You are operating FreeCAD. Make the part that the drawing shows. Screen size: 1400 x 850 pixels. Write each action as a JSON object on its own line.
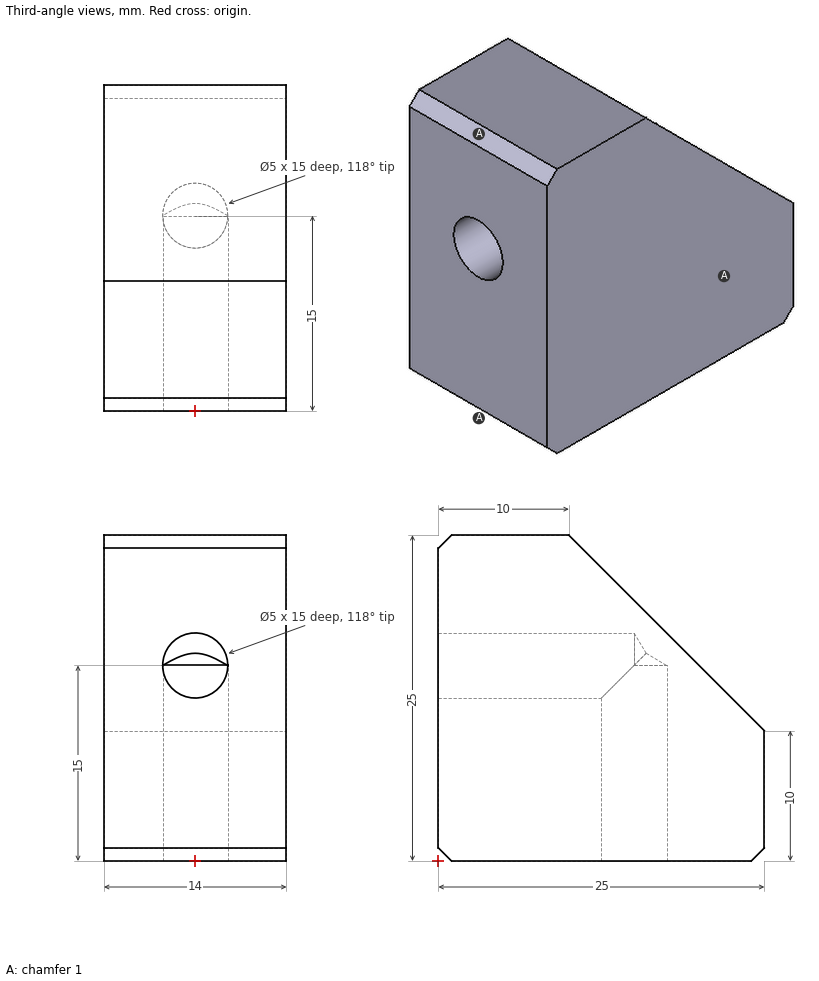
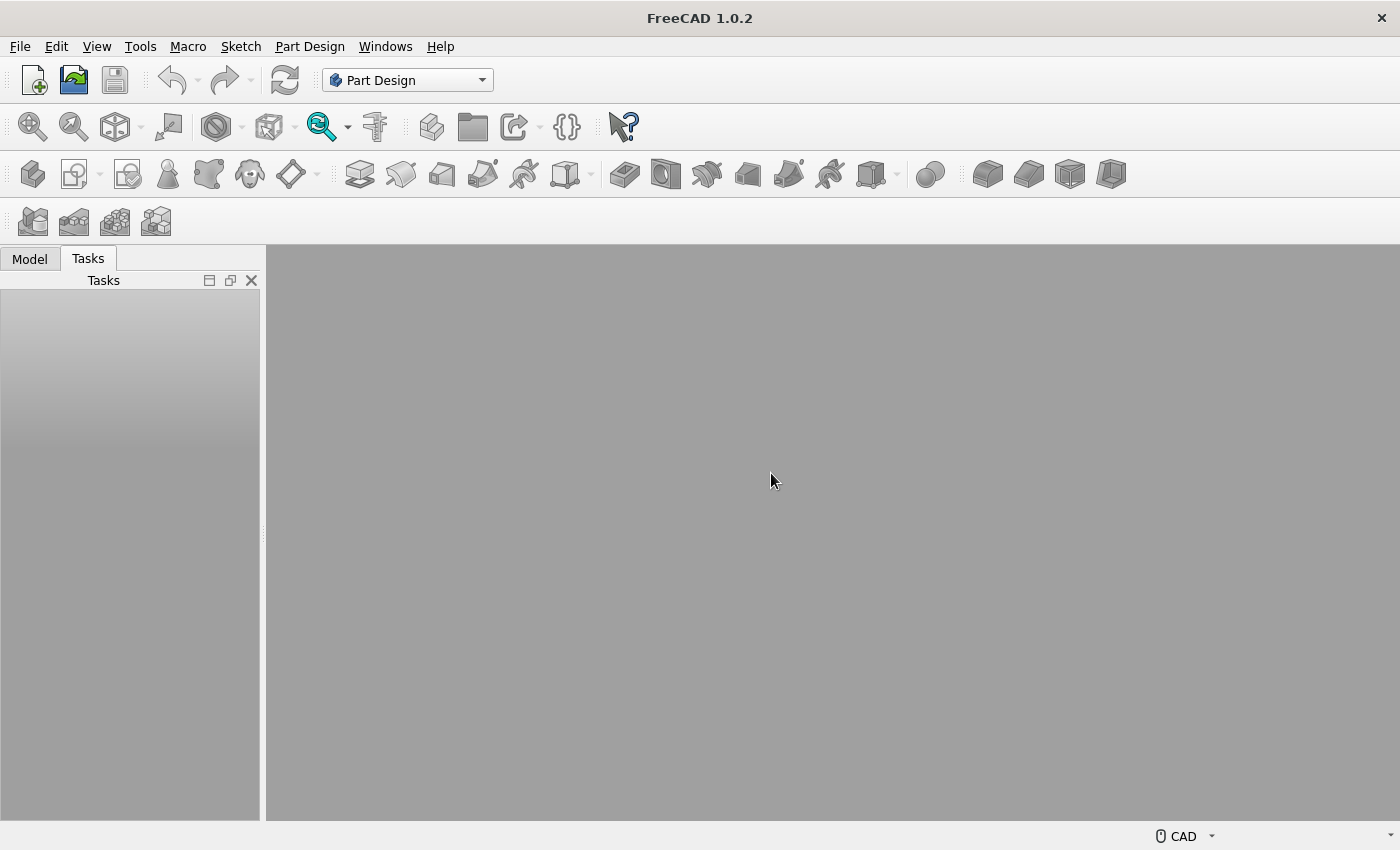
{"action": "left_click", "coordinate": [33, 80]}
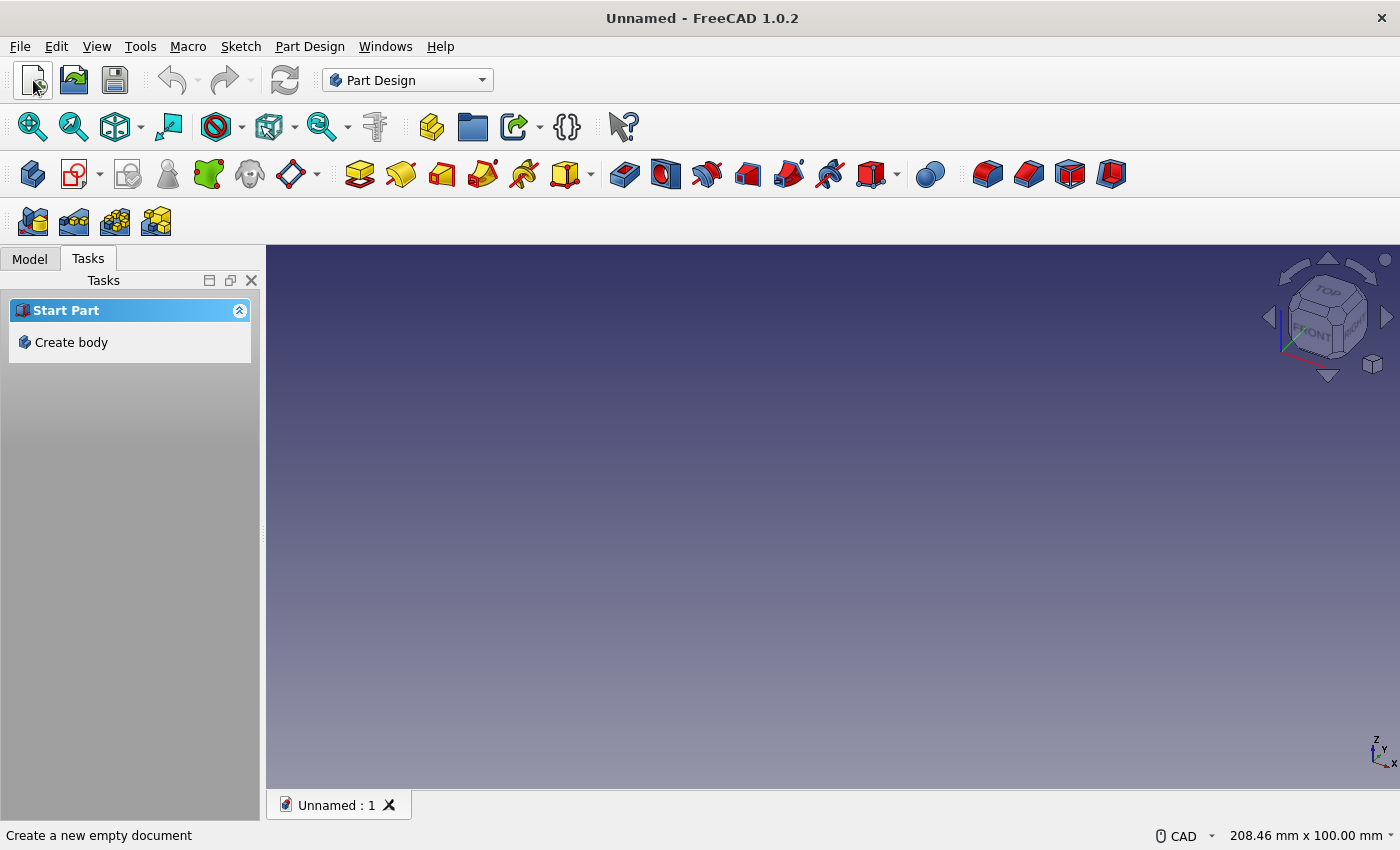
{"action": "left_click", "coordinate": [74, 174]}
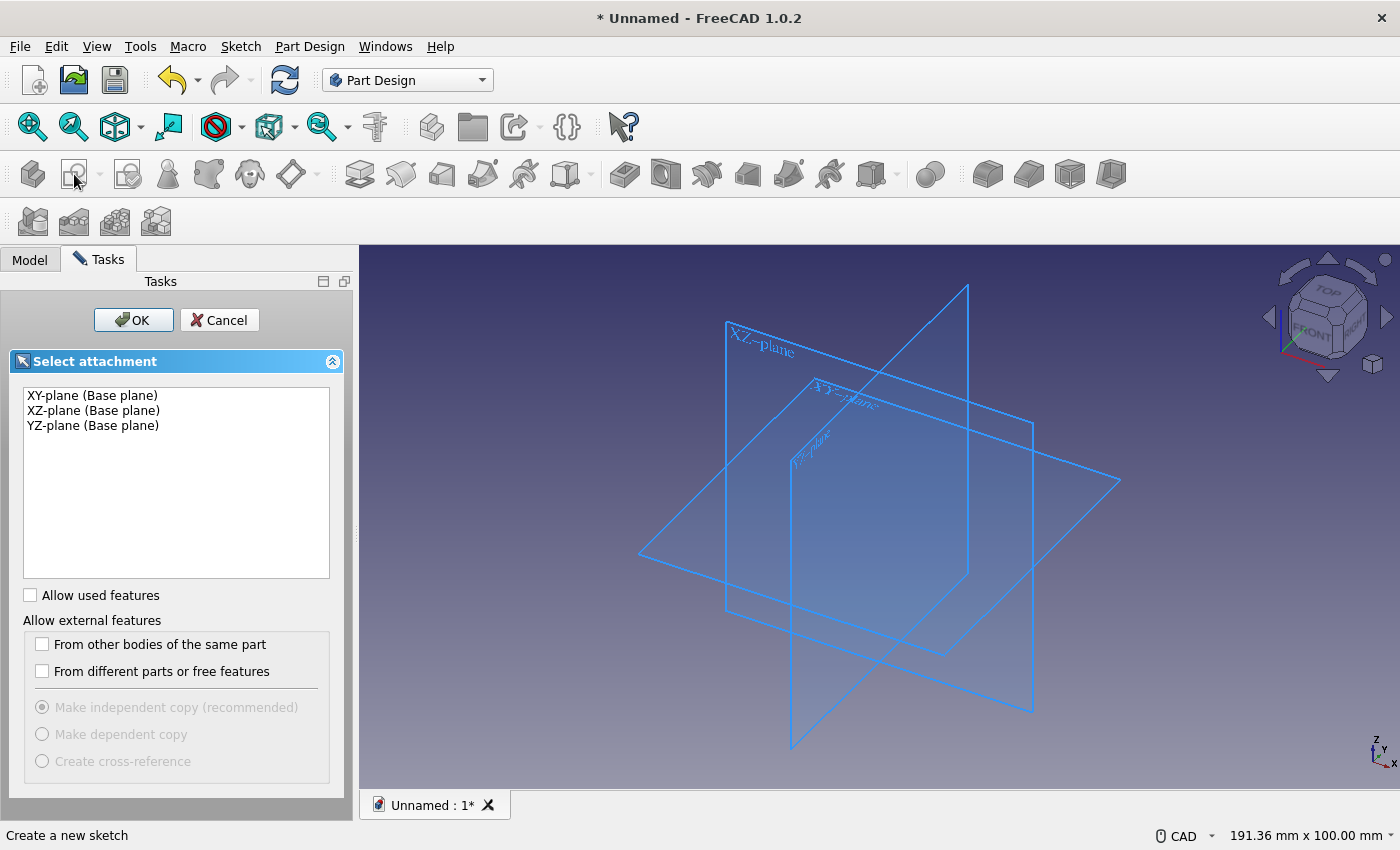
{"action": "left_click", "coordinate": [84, 426]}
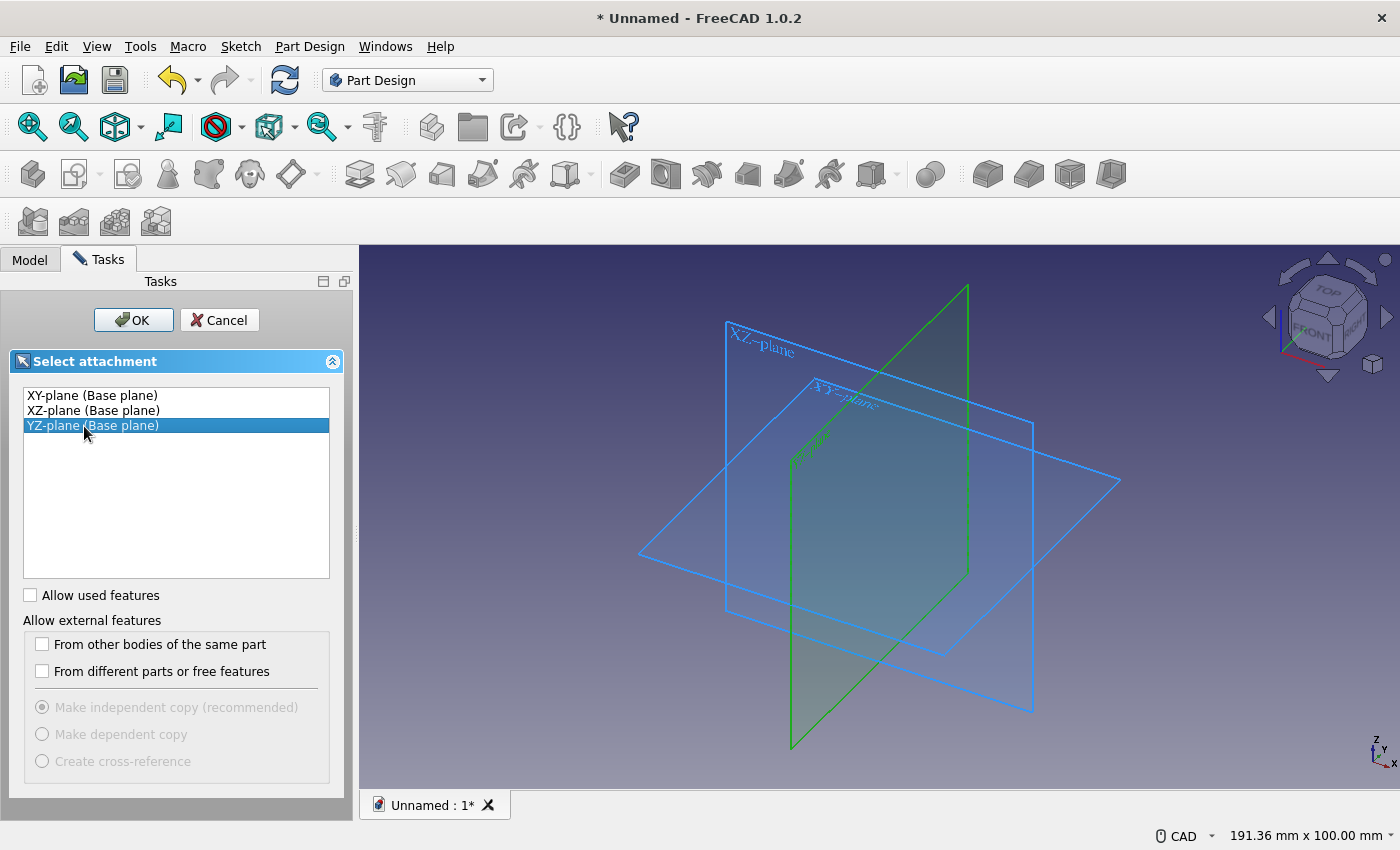
{"action": "left_click", "coordinate": [134, 320]}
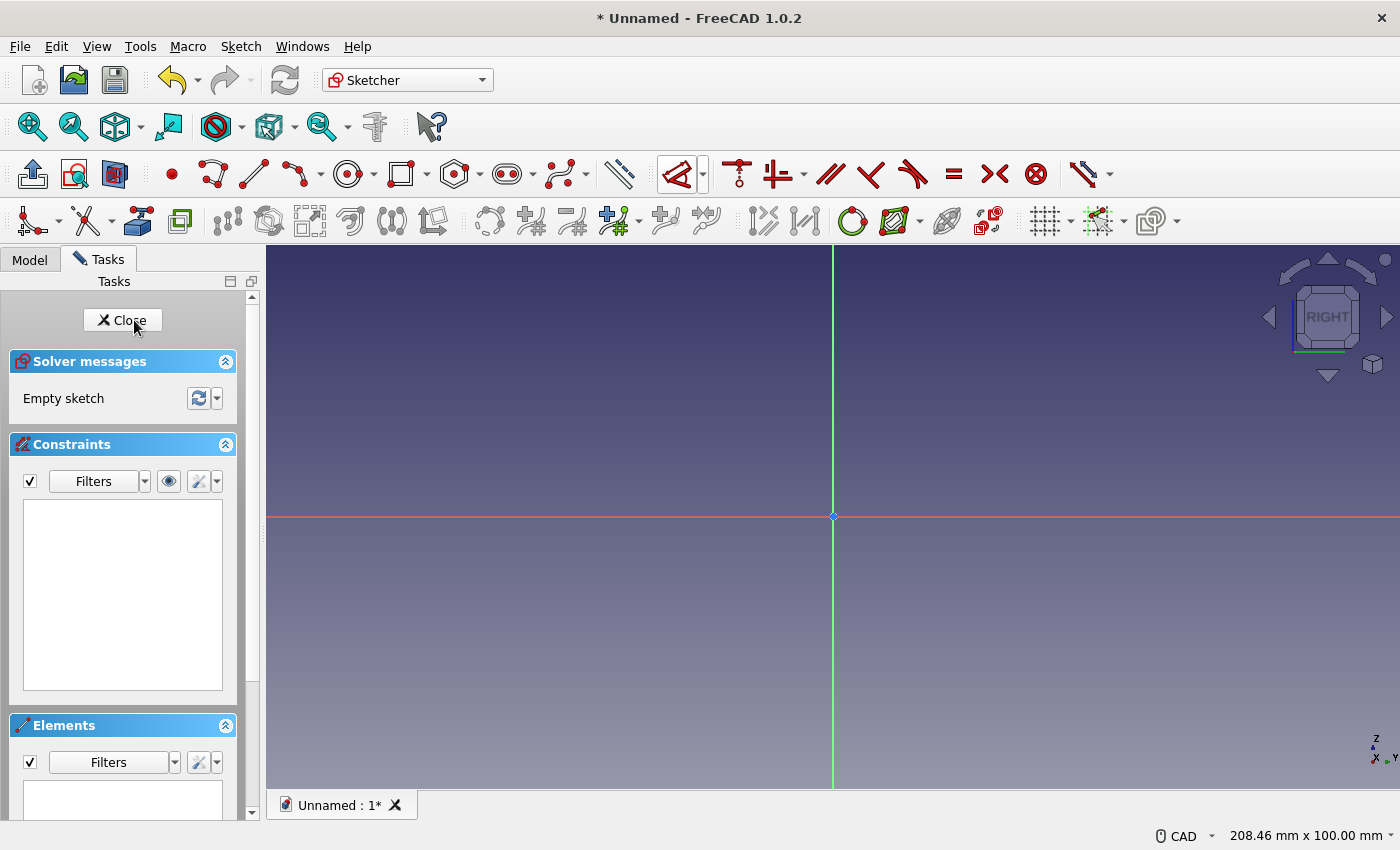
{"action": "scroll", "coordinate": [980, 409], "scroll_direction": "up", "scroll_amount": 5}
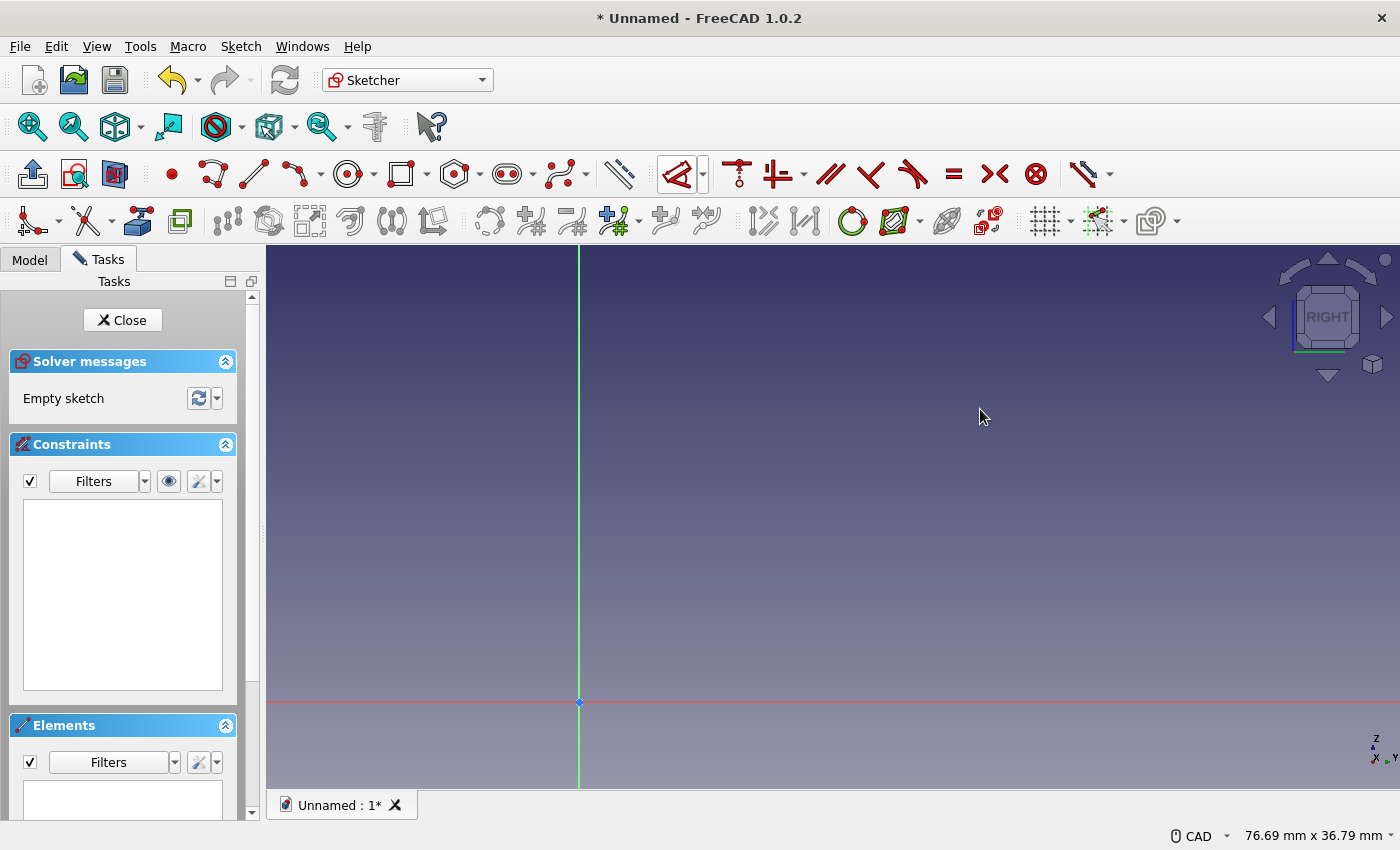
{"action": "left_click", "coordinate": [213, 174]}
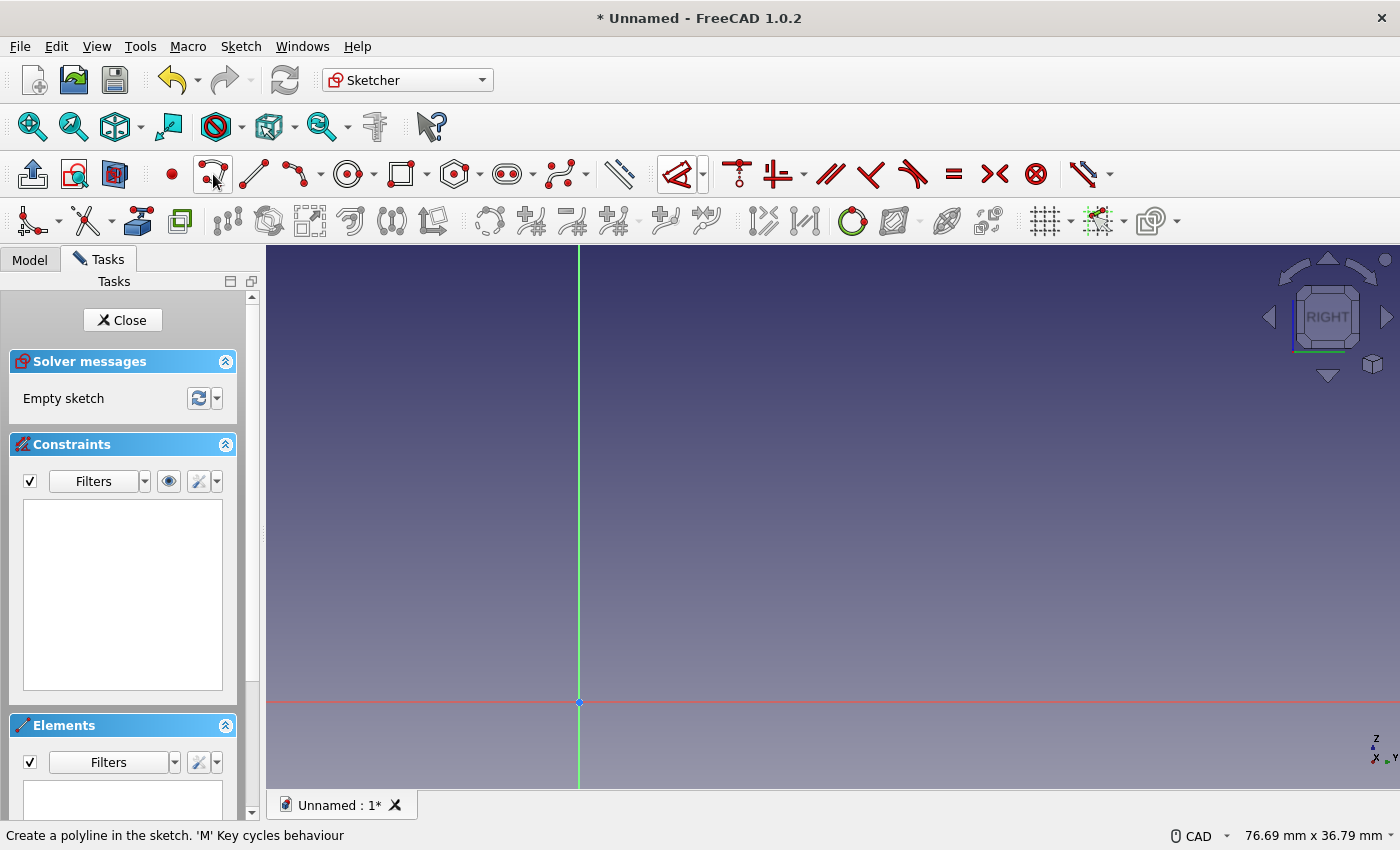
{"action": "left_click", "coordinate": [579, 702]}
{"action": "left_click", "coordinate": [949, 693]}
{"action": "left_click", "coordinate": [949, 554]}
{"action": "left_click", "coordinate": [727, 332]}
{"action": "left_click", "coordinate": [588, 332]}
{"action": "left_click", "coordinate": [579, 702]}
{"action": "key", "text": "Escape"}
{"action": "key", "text": "Escape"}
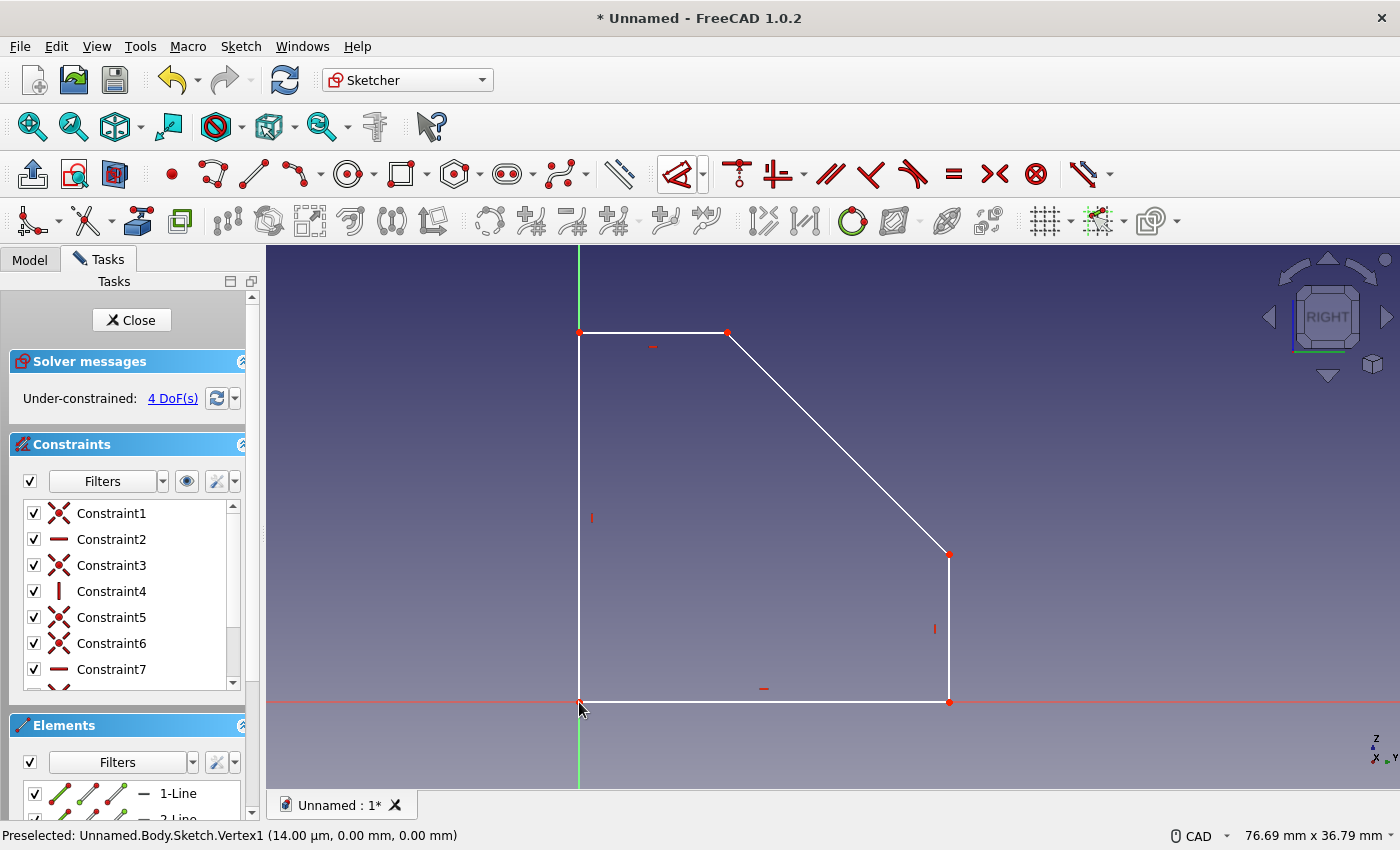
{"action": "left_click", "coordinate": [676, 174]}